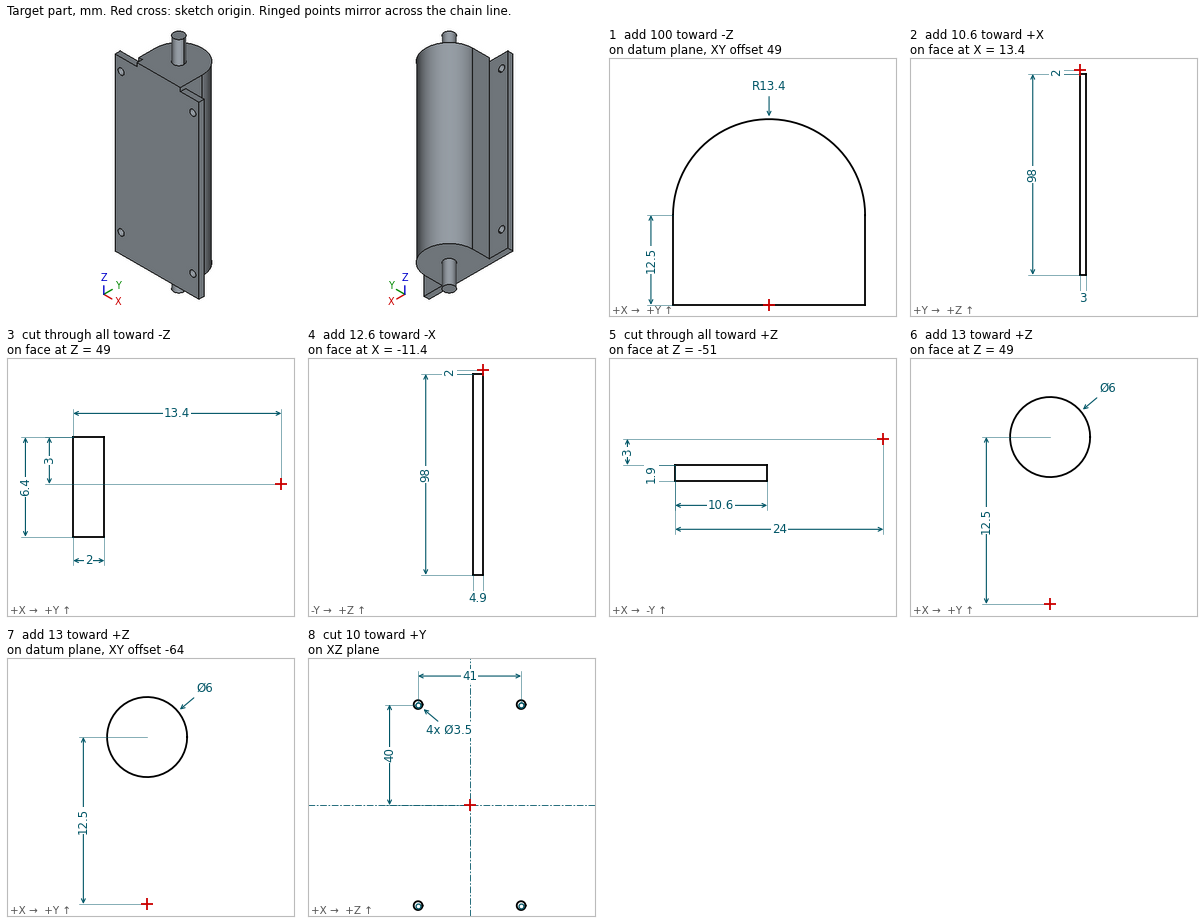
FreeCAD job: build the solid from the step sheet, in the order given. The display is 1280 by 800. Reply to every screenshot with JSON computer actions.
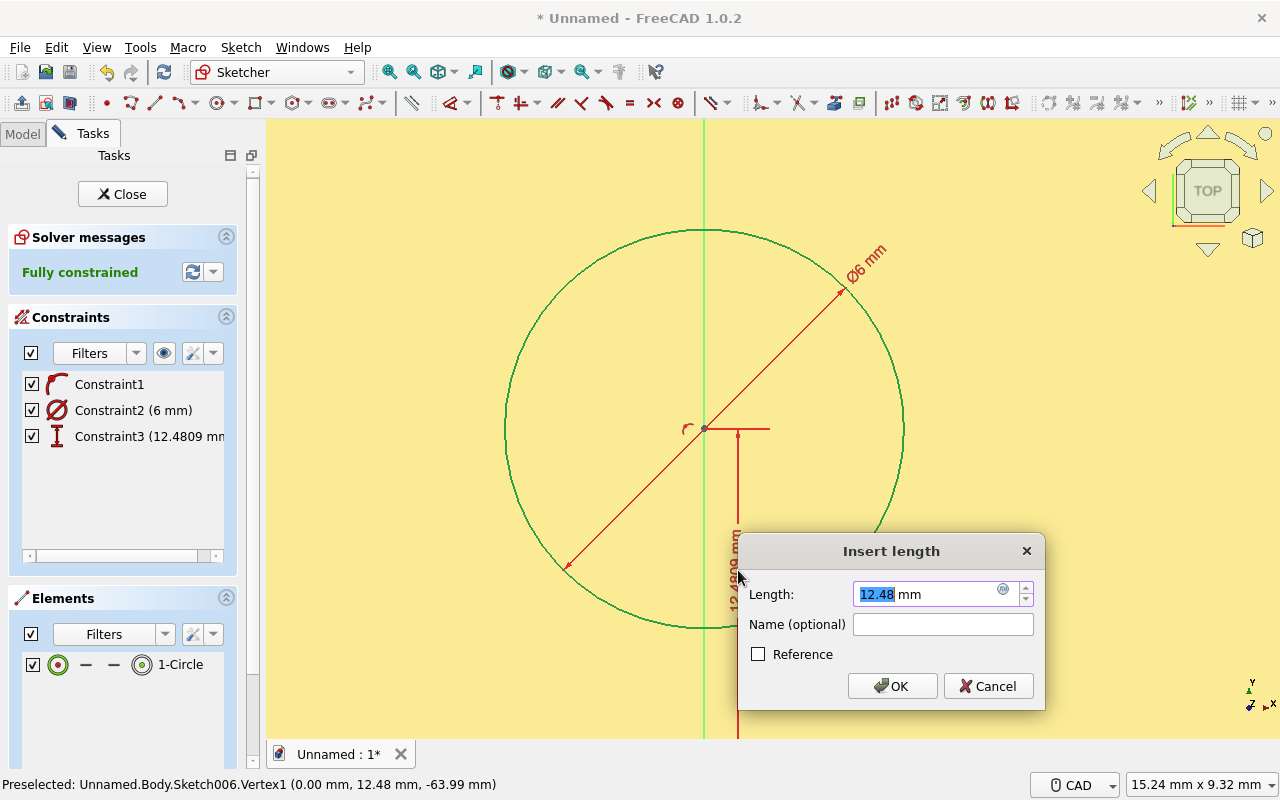
{"action": "type", "text": "12.5"}
{"action": "key", "text": "Return"}
{"action": "key", "text": "Escape"}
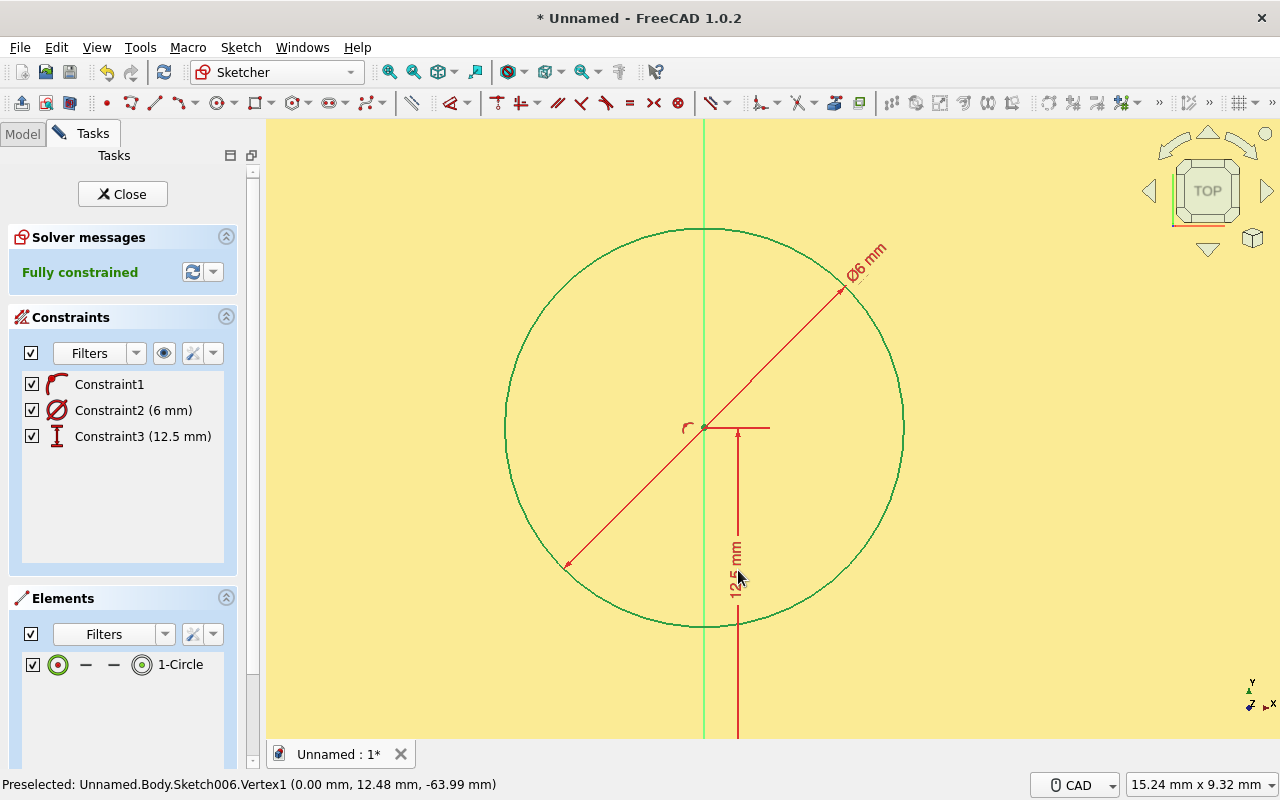
{"action": "left_click", "coordinate": [123, 194]}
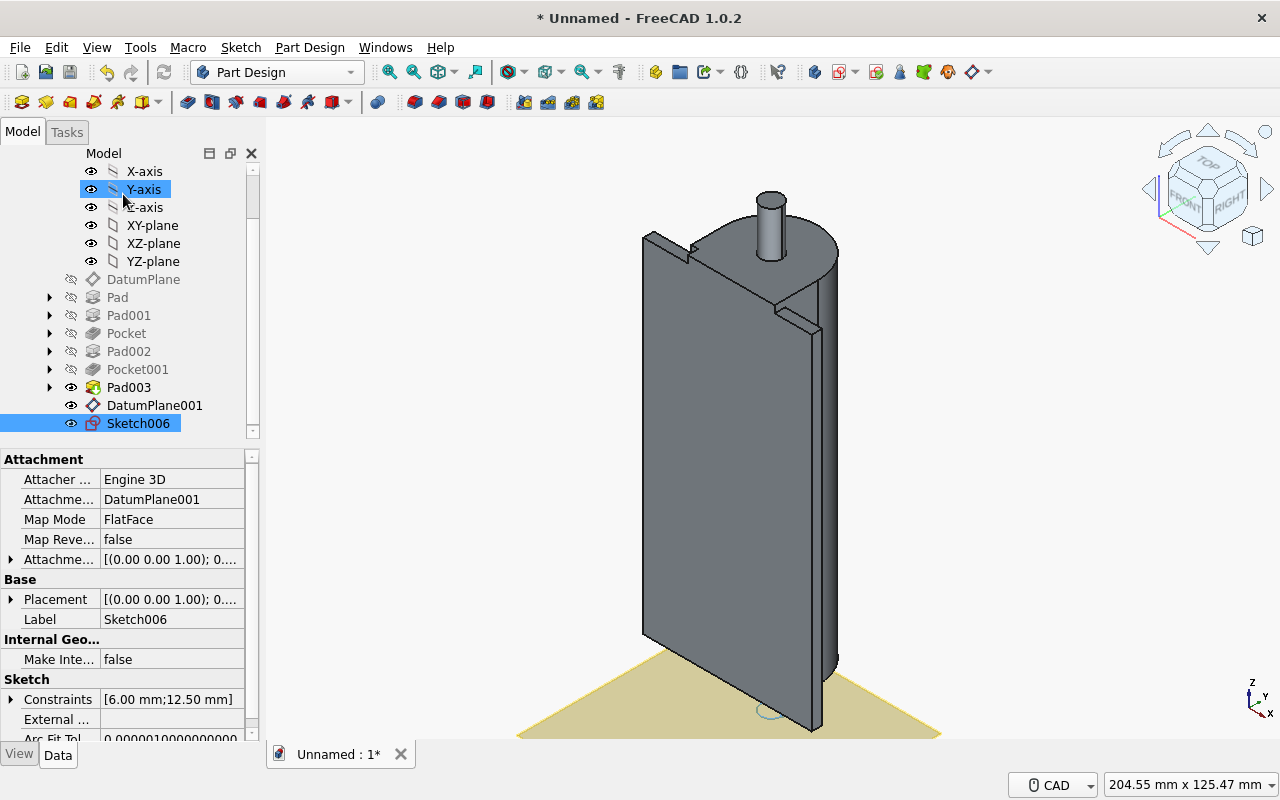
{"action": "left_click", "coordinate": [22, 102]}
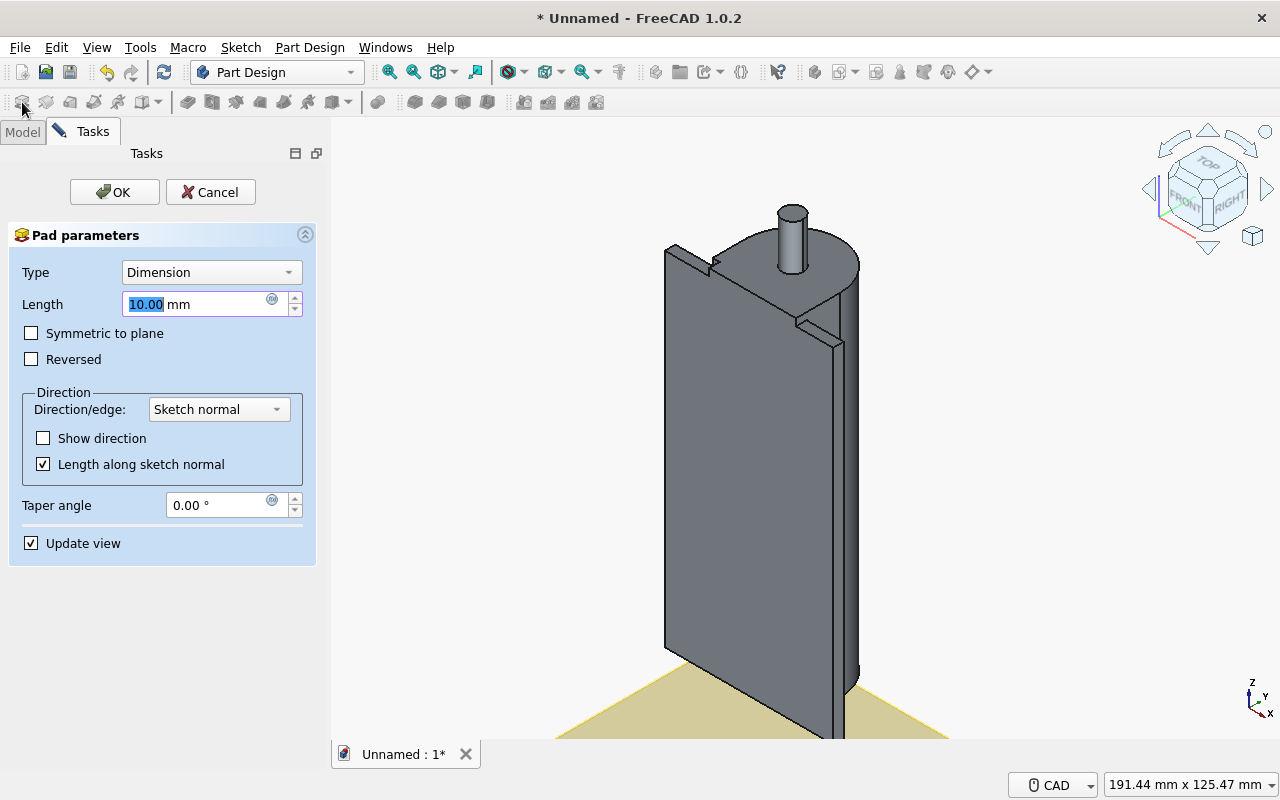
{"action": "type", "text": "13"}
{"action": "key", "text": "Tab"}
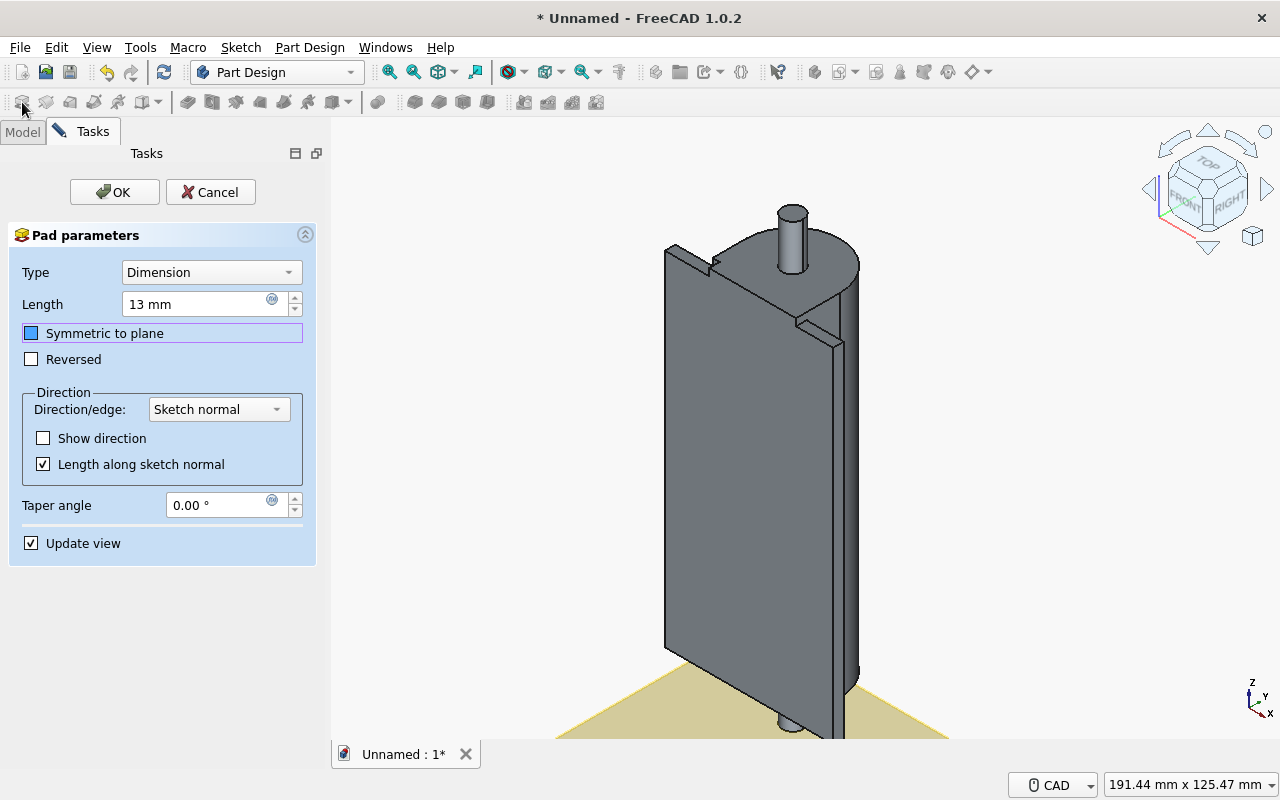
{"action": "left_click", "coordinate": [115, 192]}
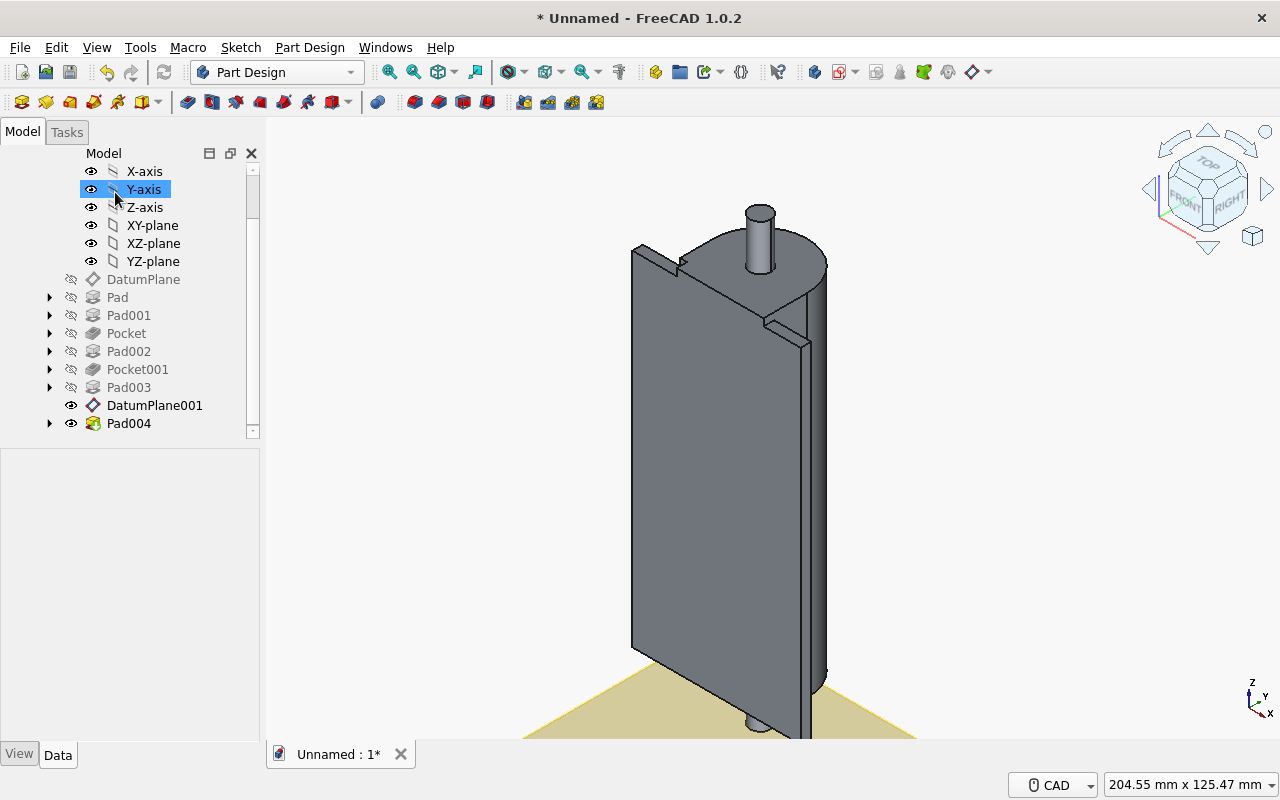
{"action": "left_click", "coordinate": [116, 405]}
{"action": "key", "text": "space"}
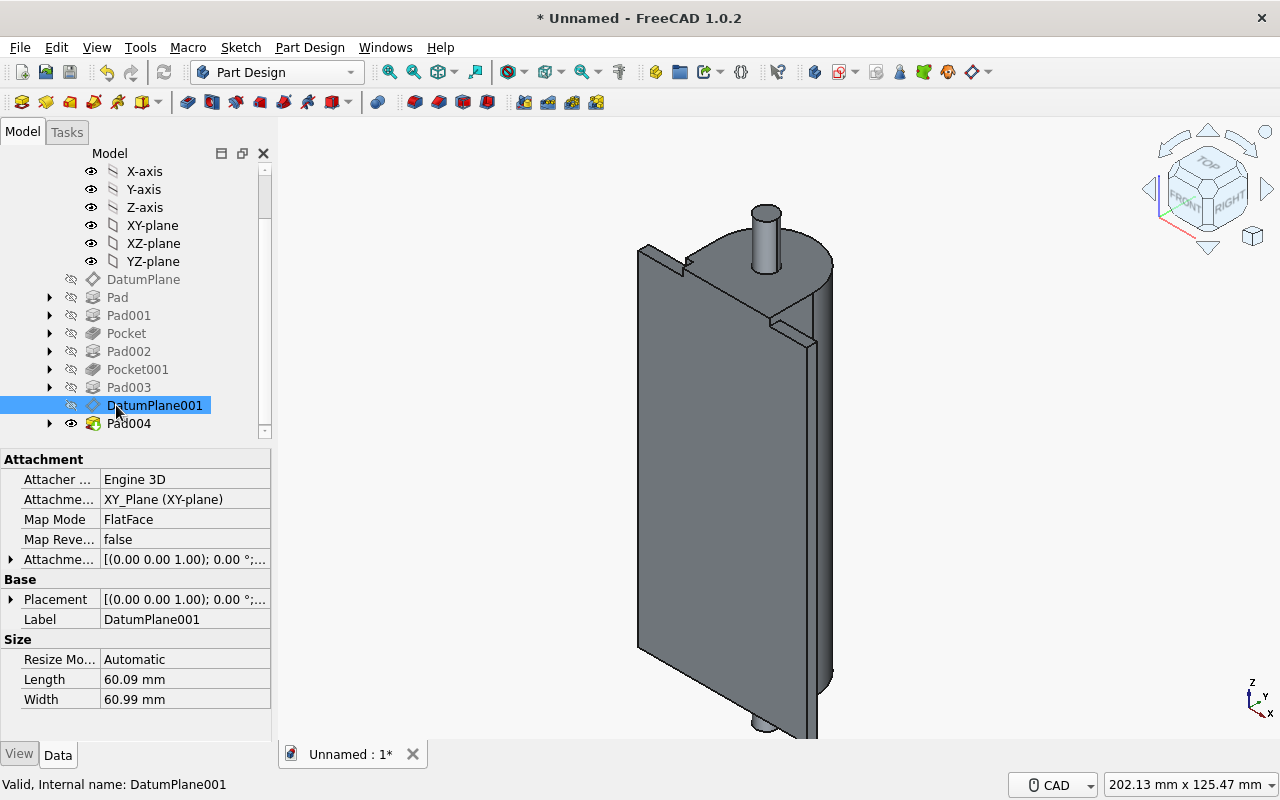
{"action": "left_click", "coordinate": [390, 72]}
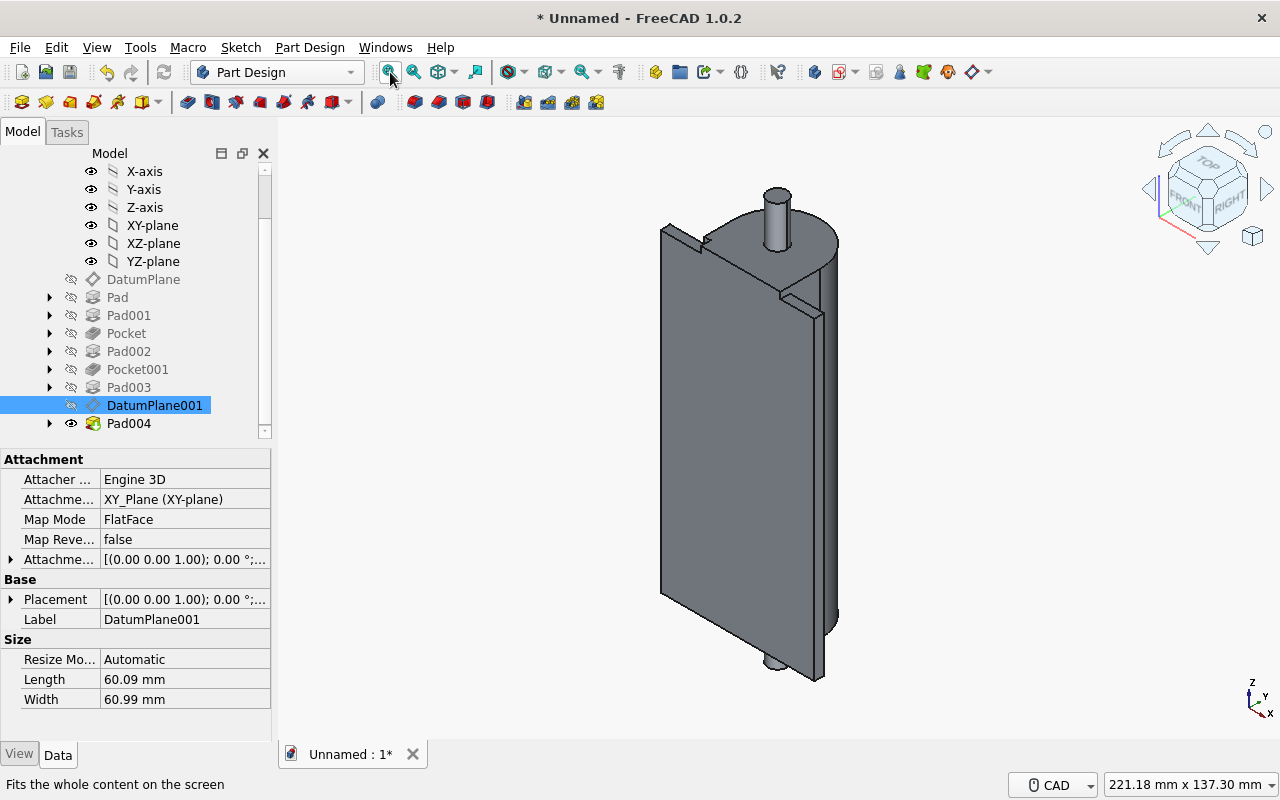
{"action": "left_click", "coordinate": [318, 699]}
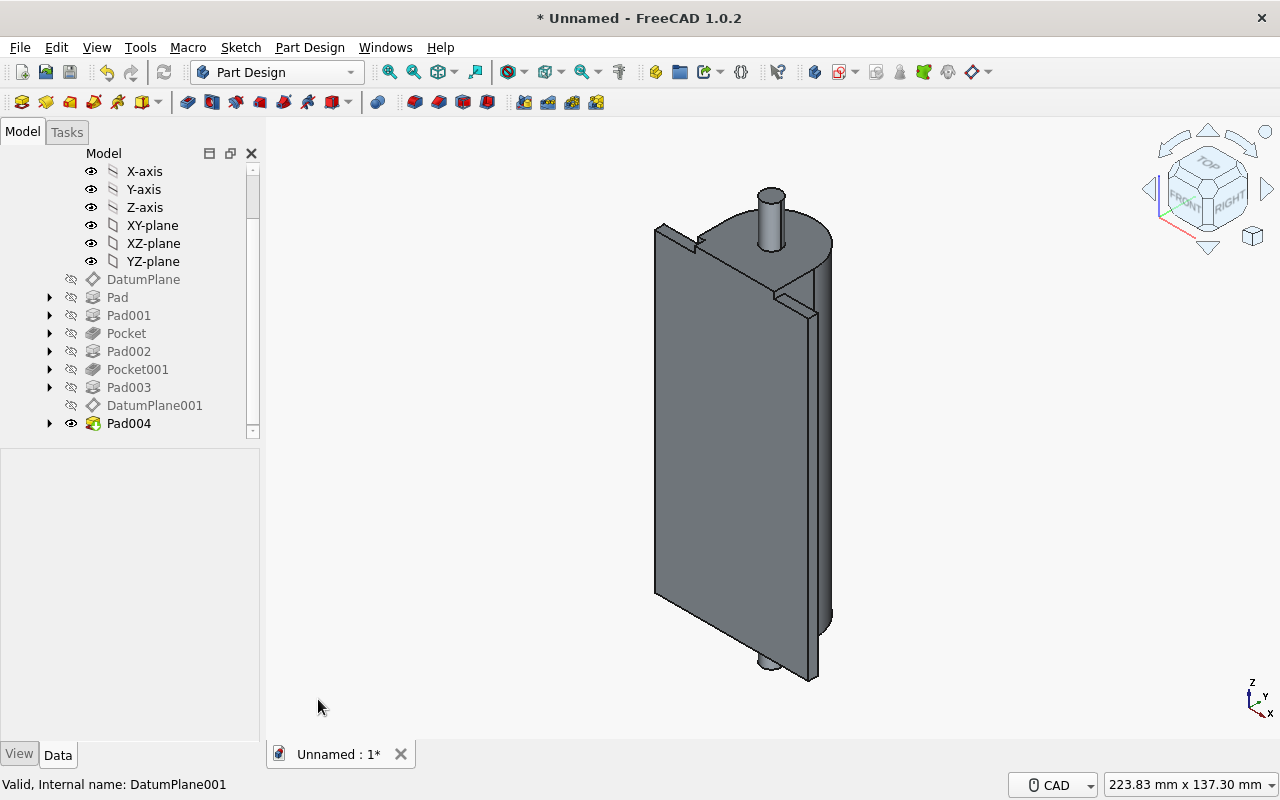
{"action": "left_click", "coordinate": [840, 72]}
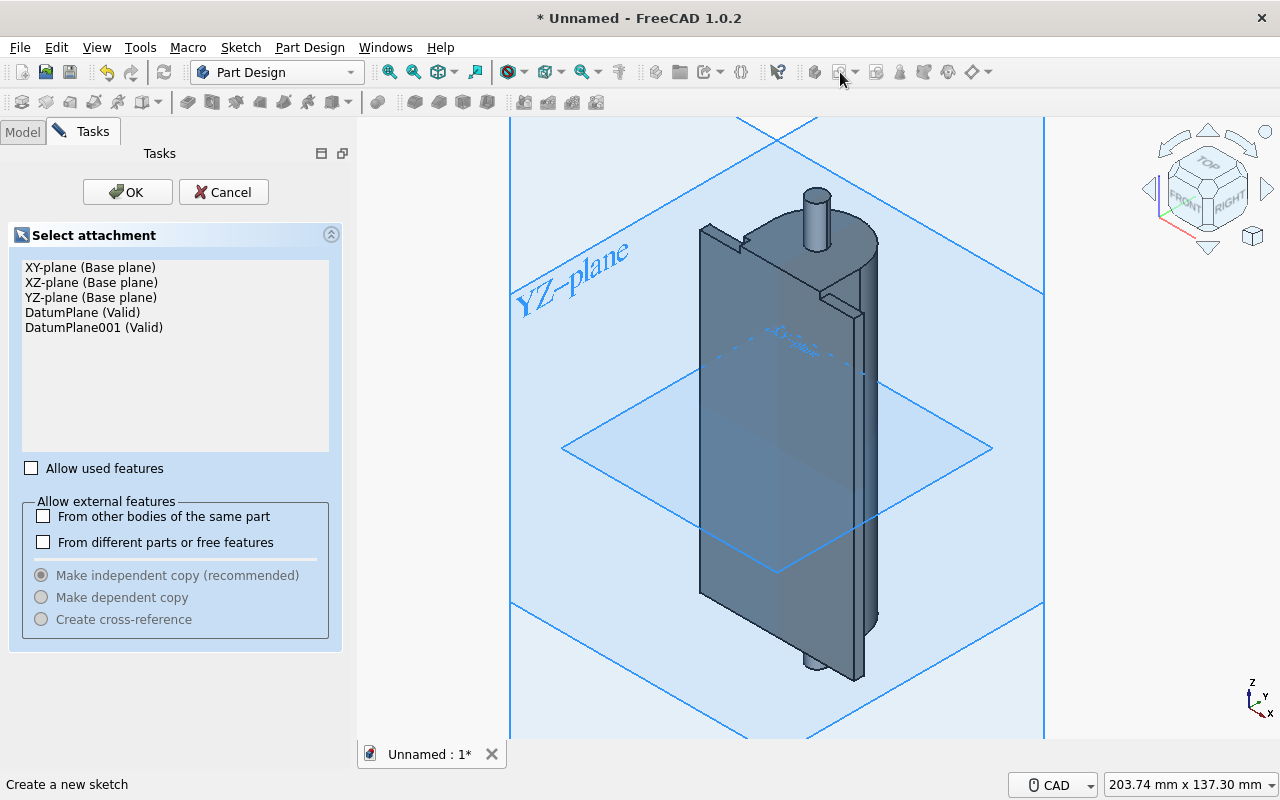
{"action": "left_click", "coordinate": [82, 282]}